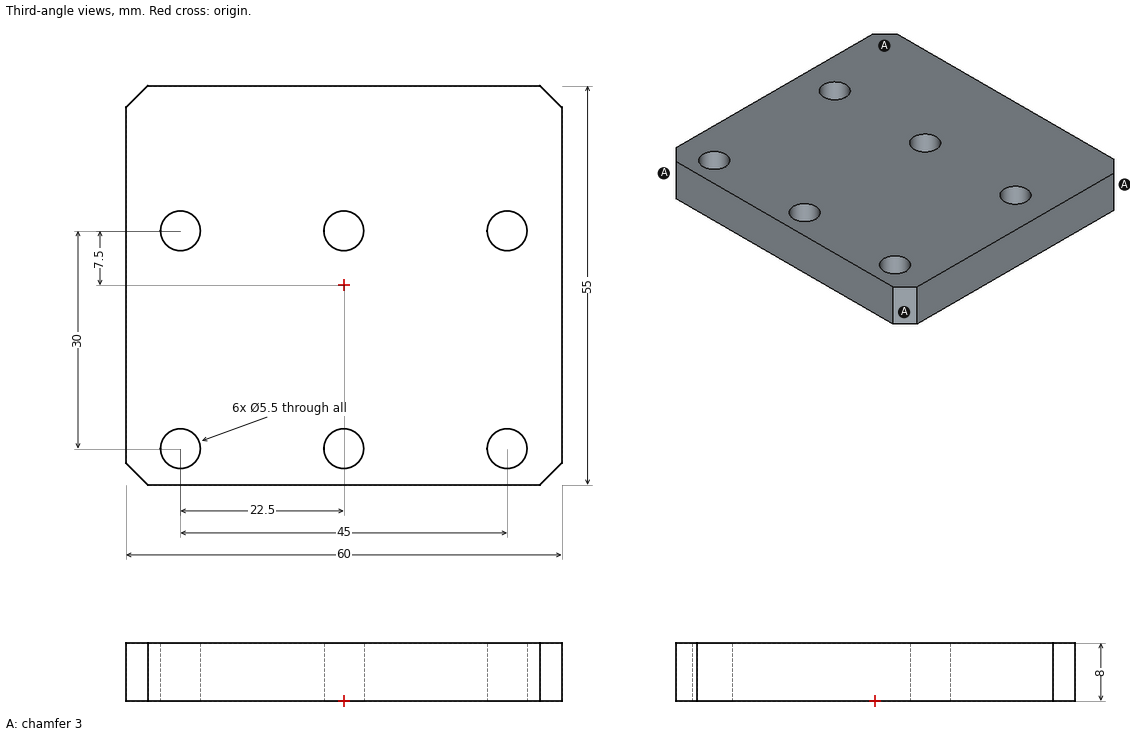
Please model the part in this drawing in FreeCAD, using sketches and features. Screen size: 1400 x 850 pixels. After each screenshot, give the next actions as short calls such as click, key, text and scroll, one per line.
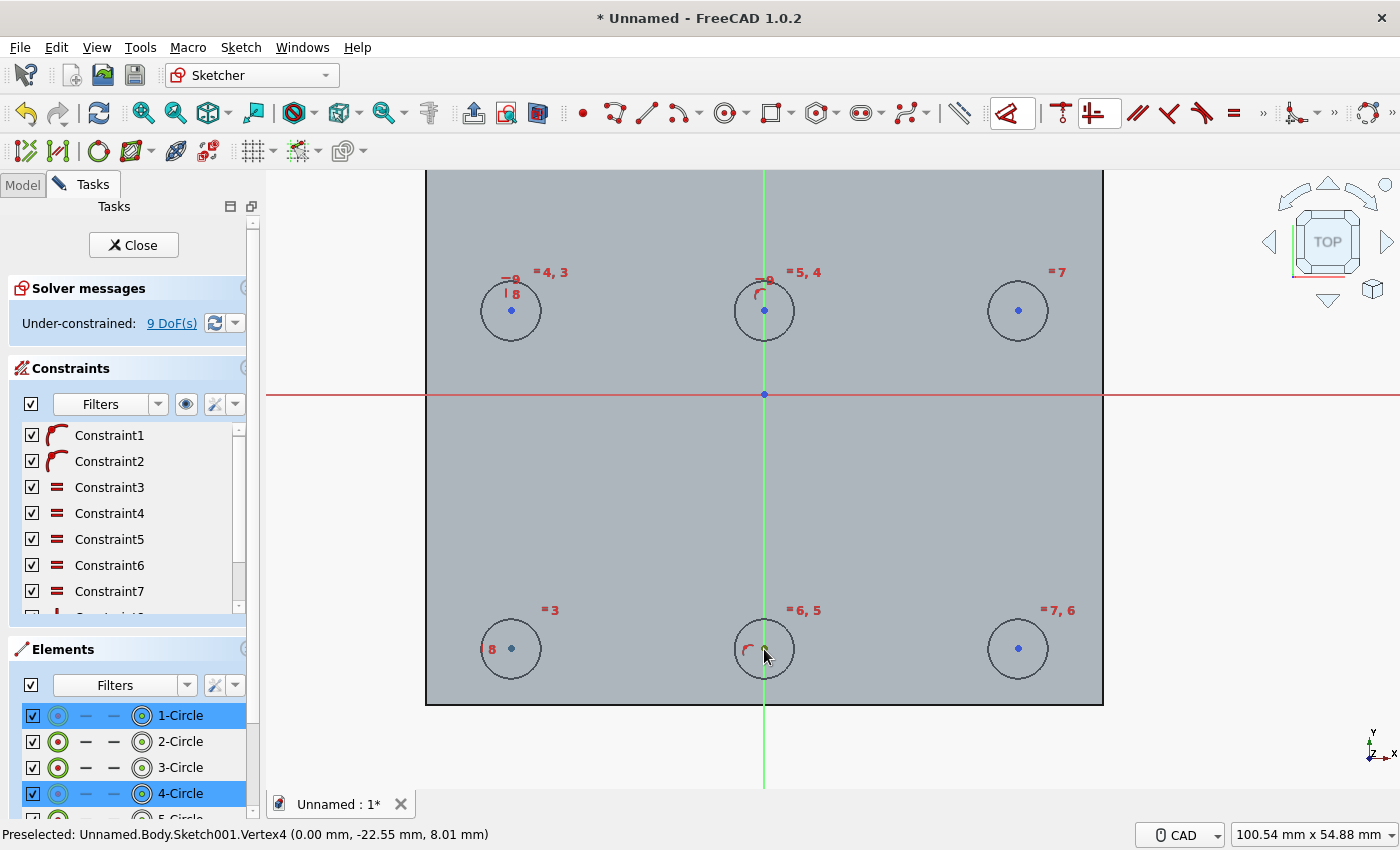
click(1116, 114)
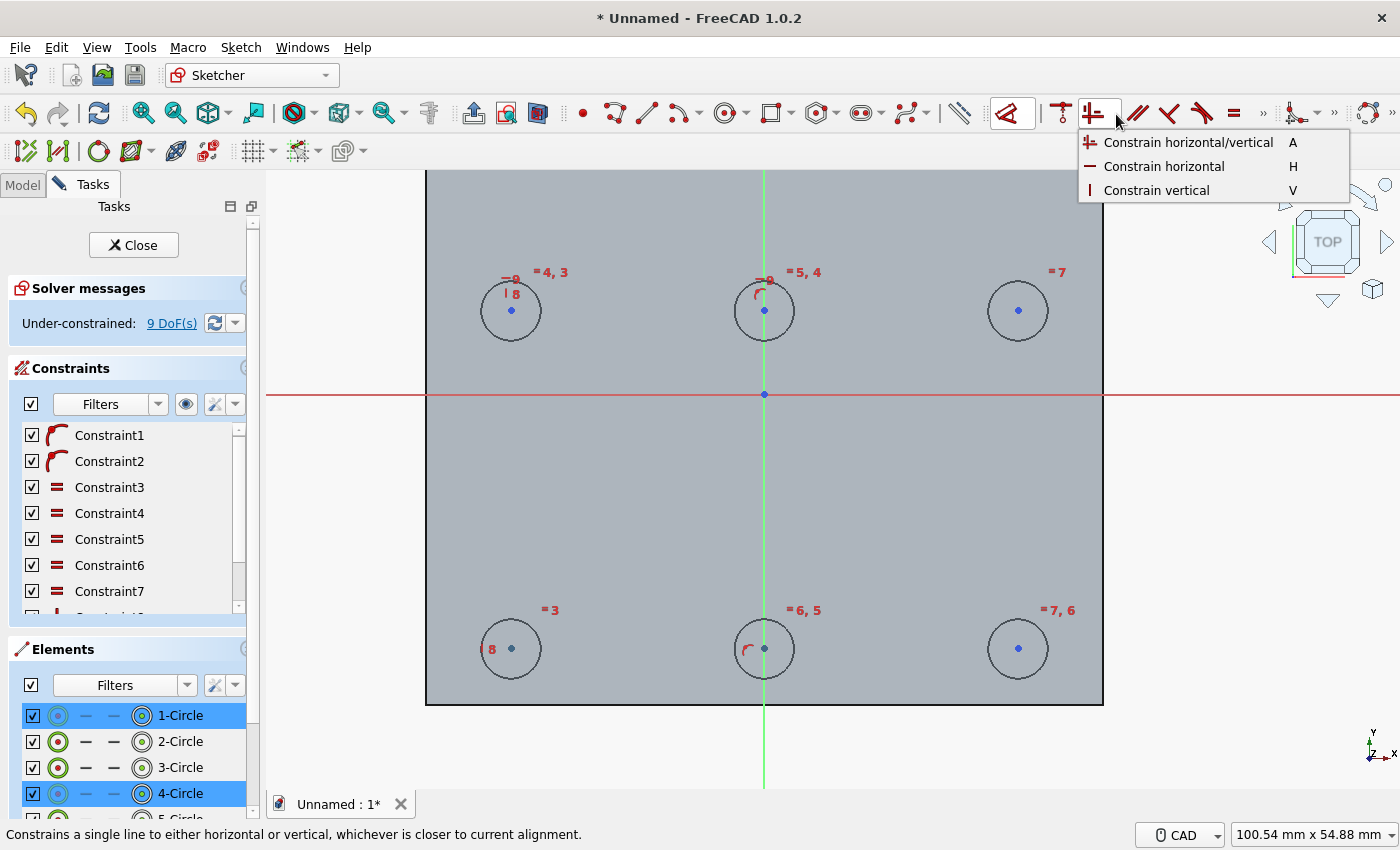
click(1214, 166)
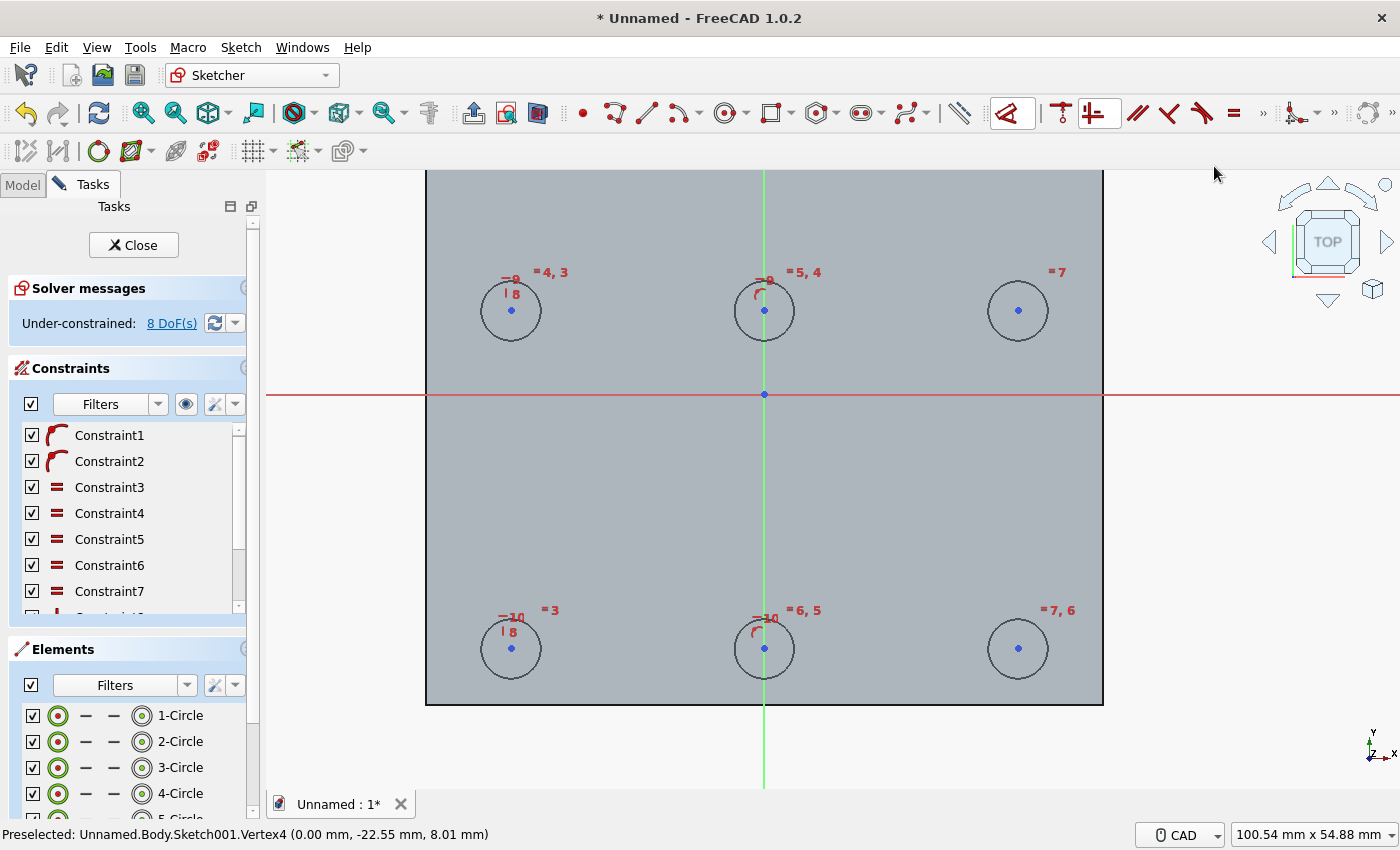
click(764, 649)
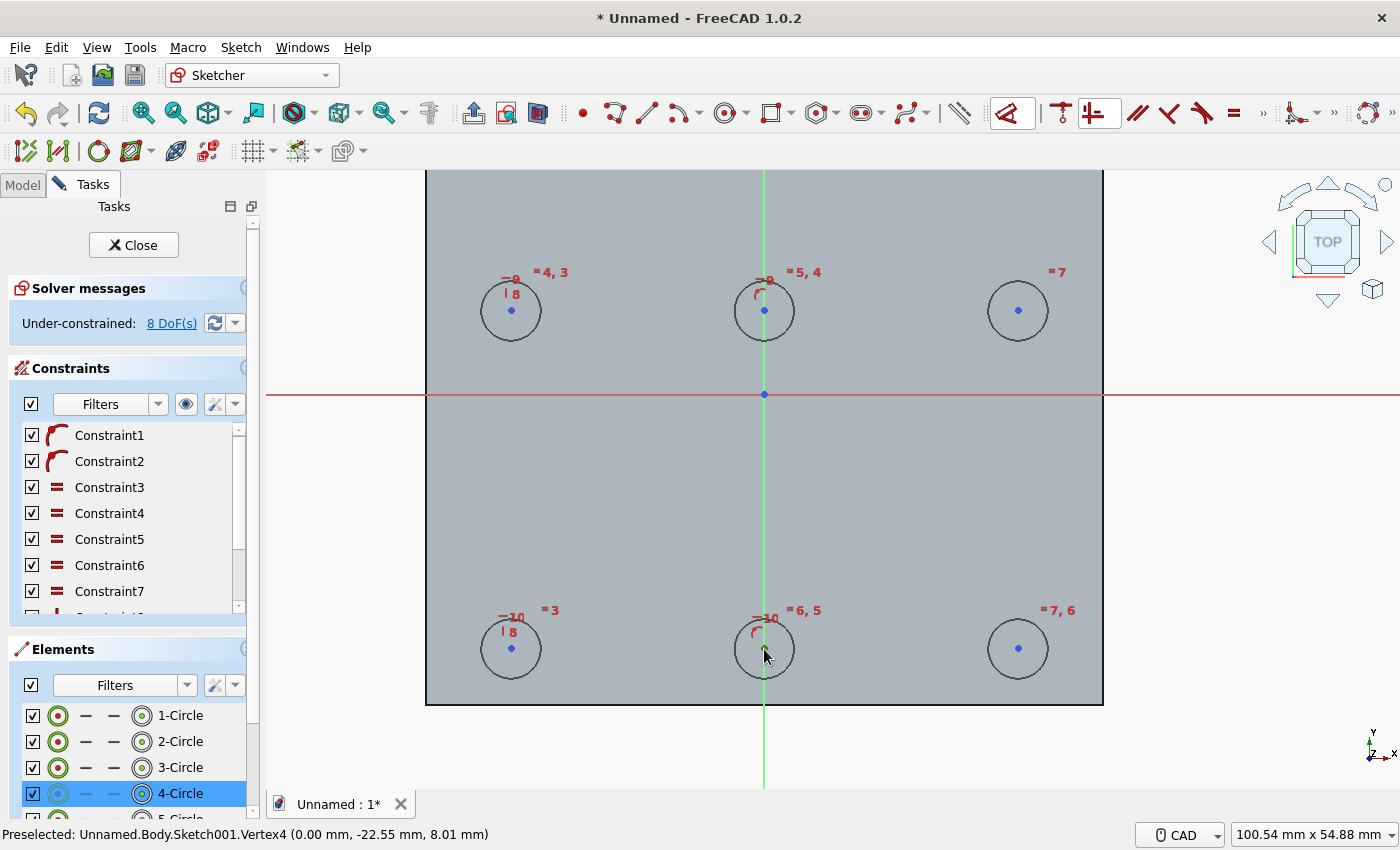
click(1018, 649)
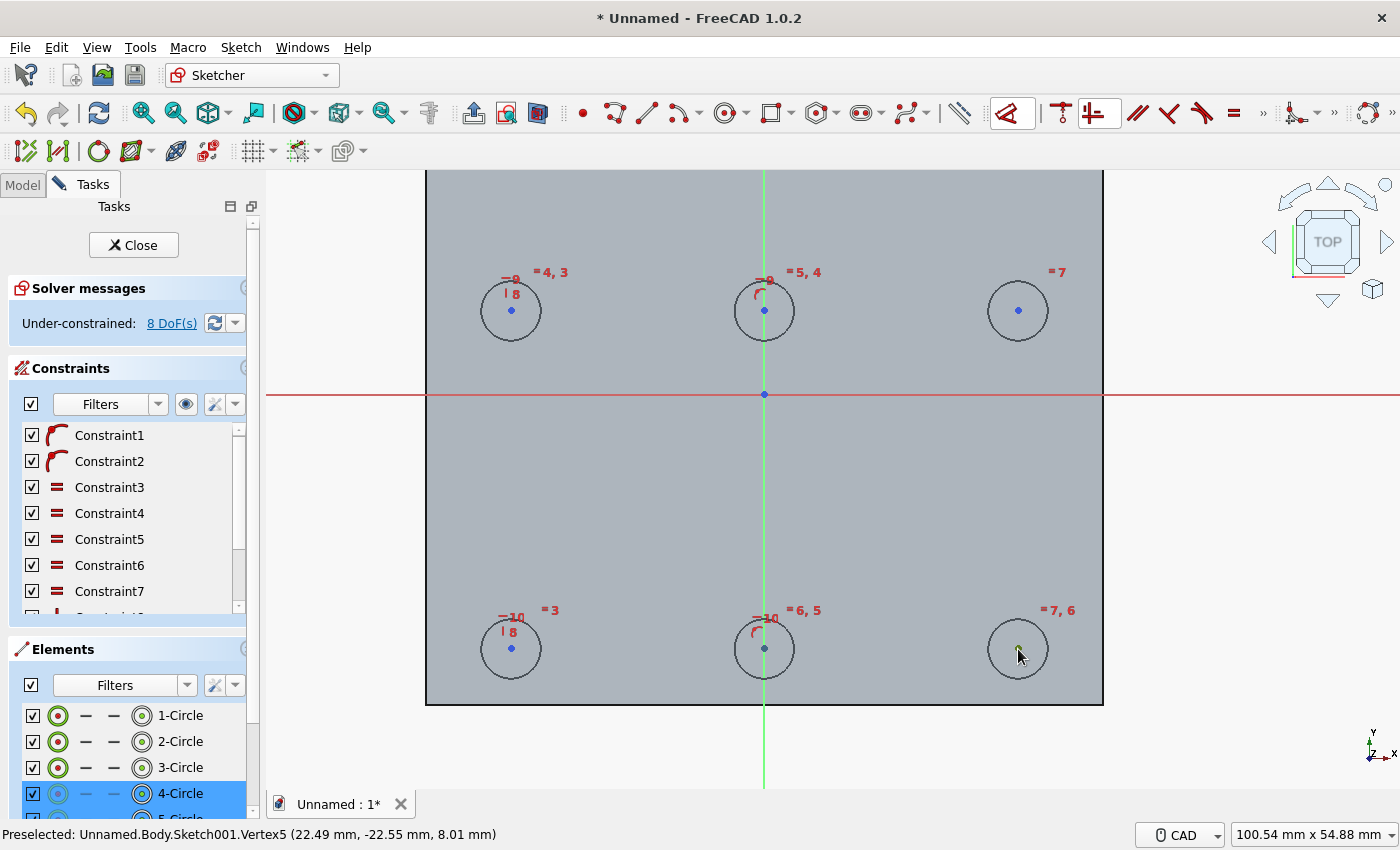
key(h)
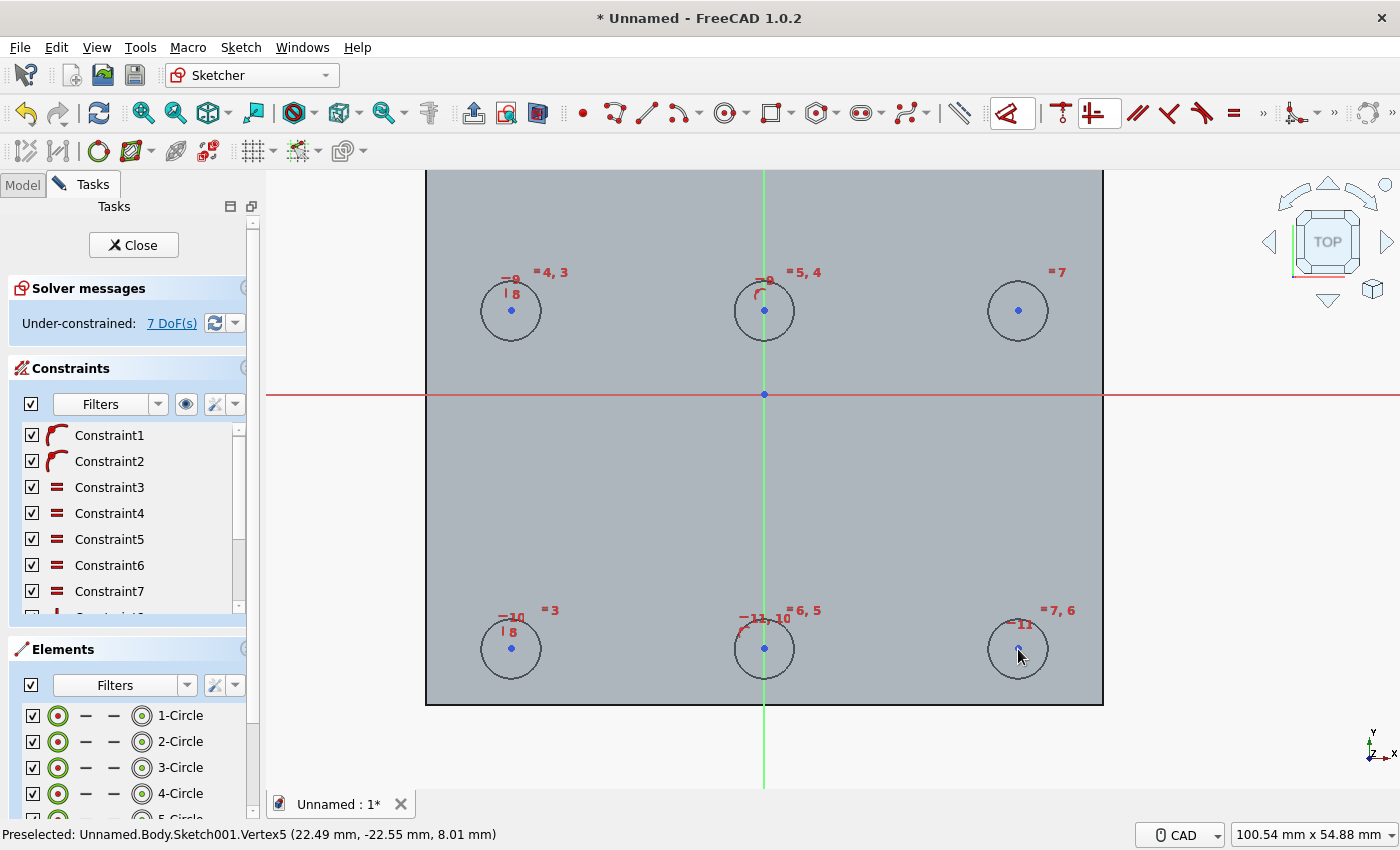
click(1018, 649)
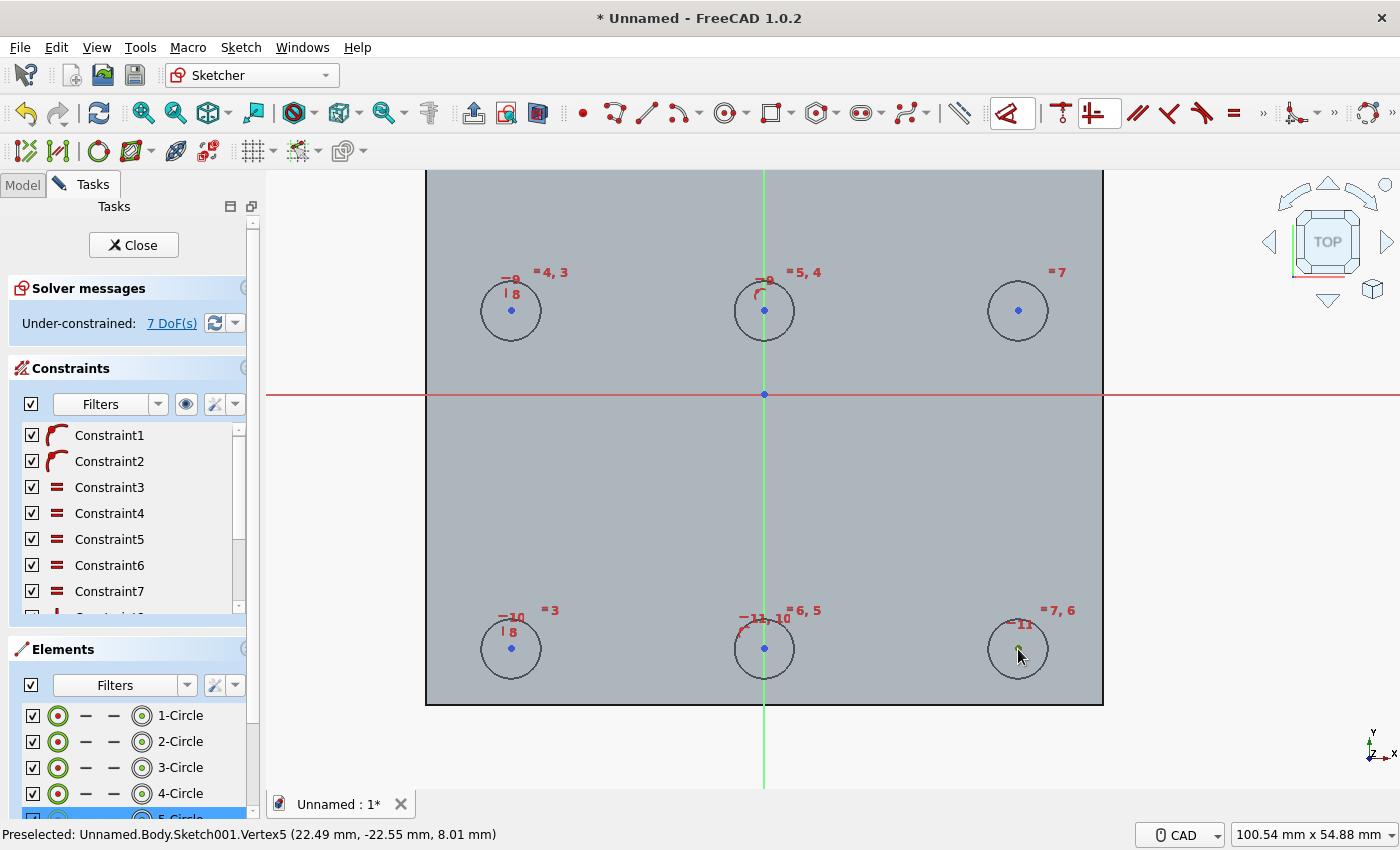
click(1018, 311)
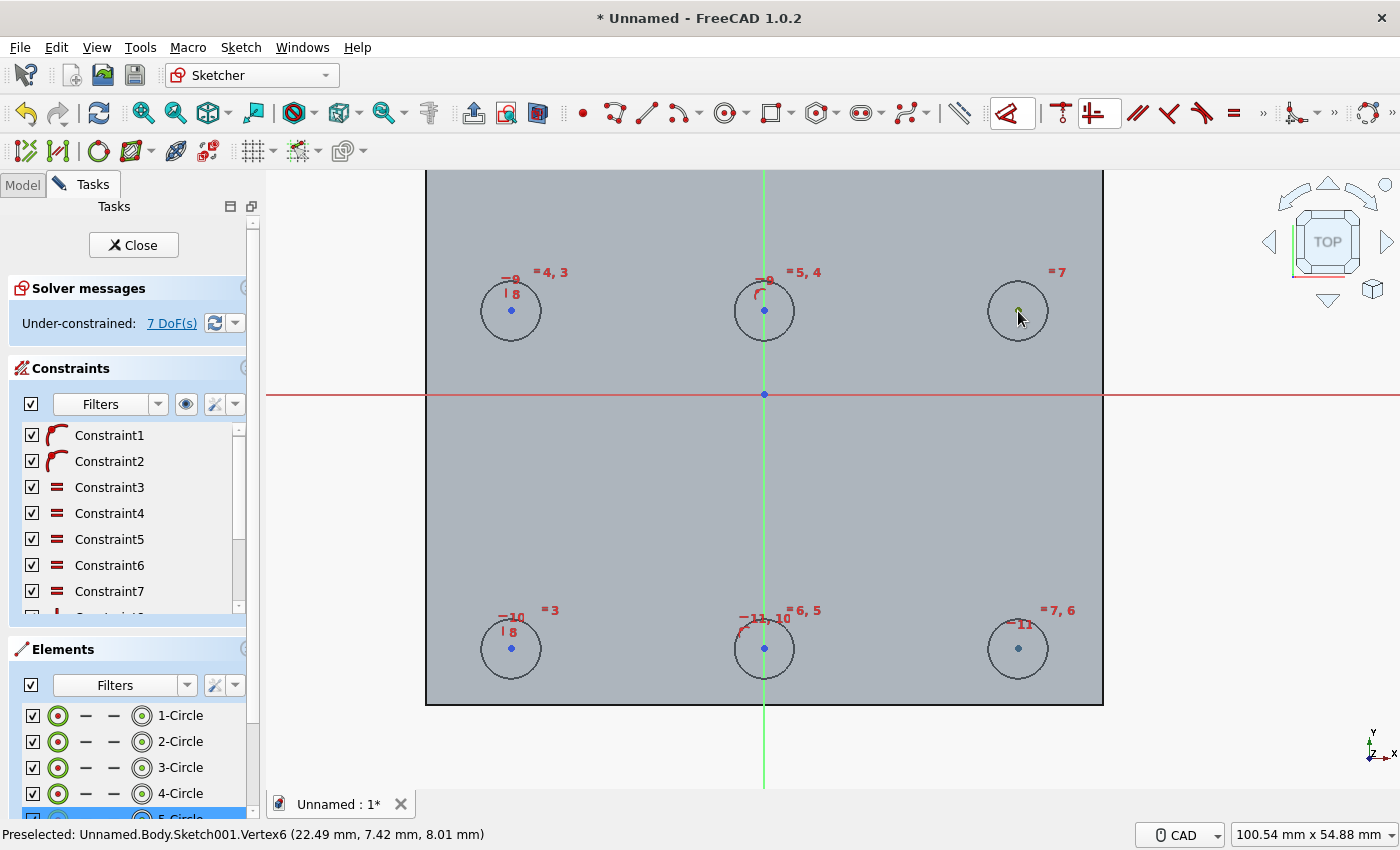
key(v)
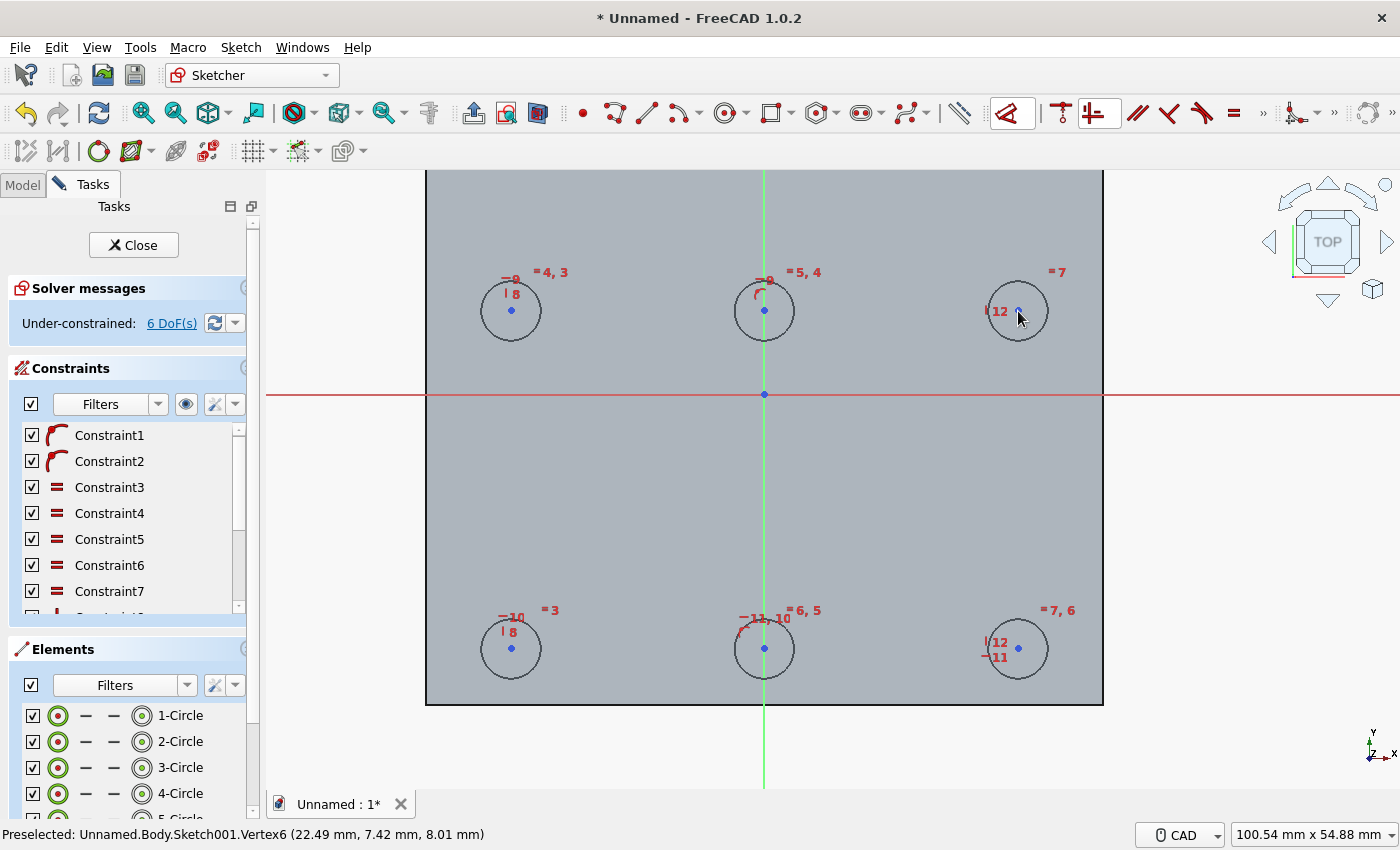
click(764, 311)